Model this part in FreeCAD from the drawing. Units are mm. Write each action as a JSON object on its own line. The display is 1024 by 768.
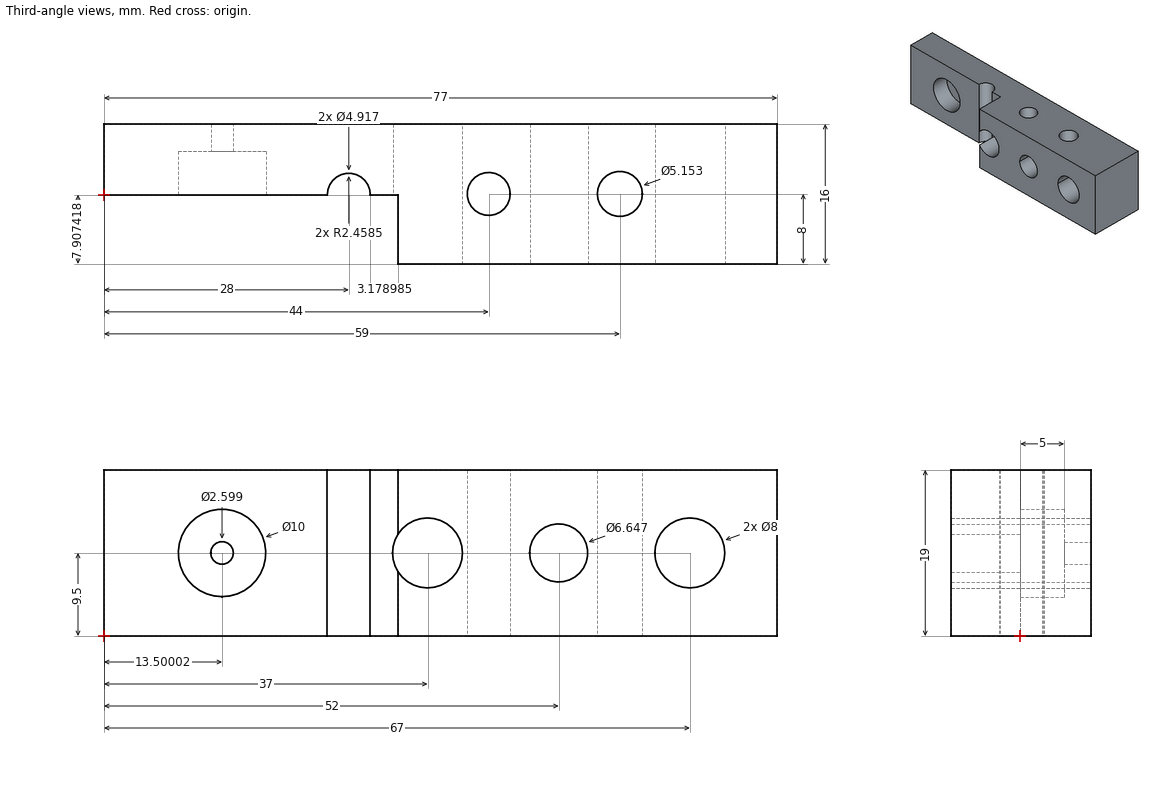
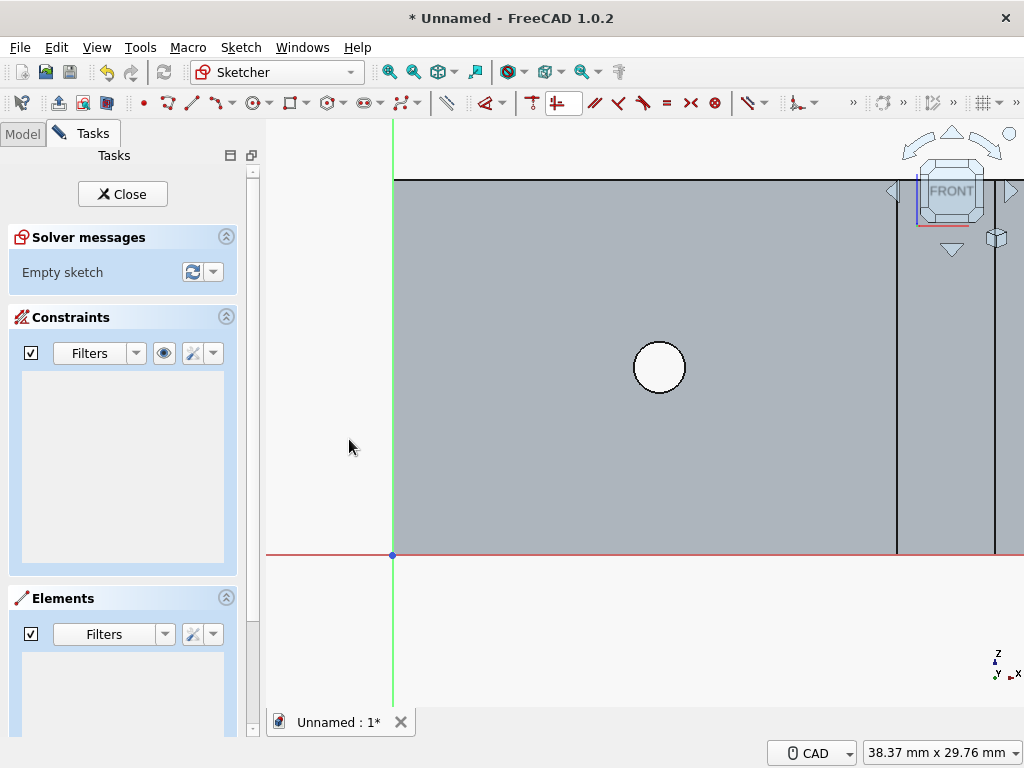
{"action": "key", "text": "g c"}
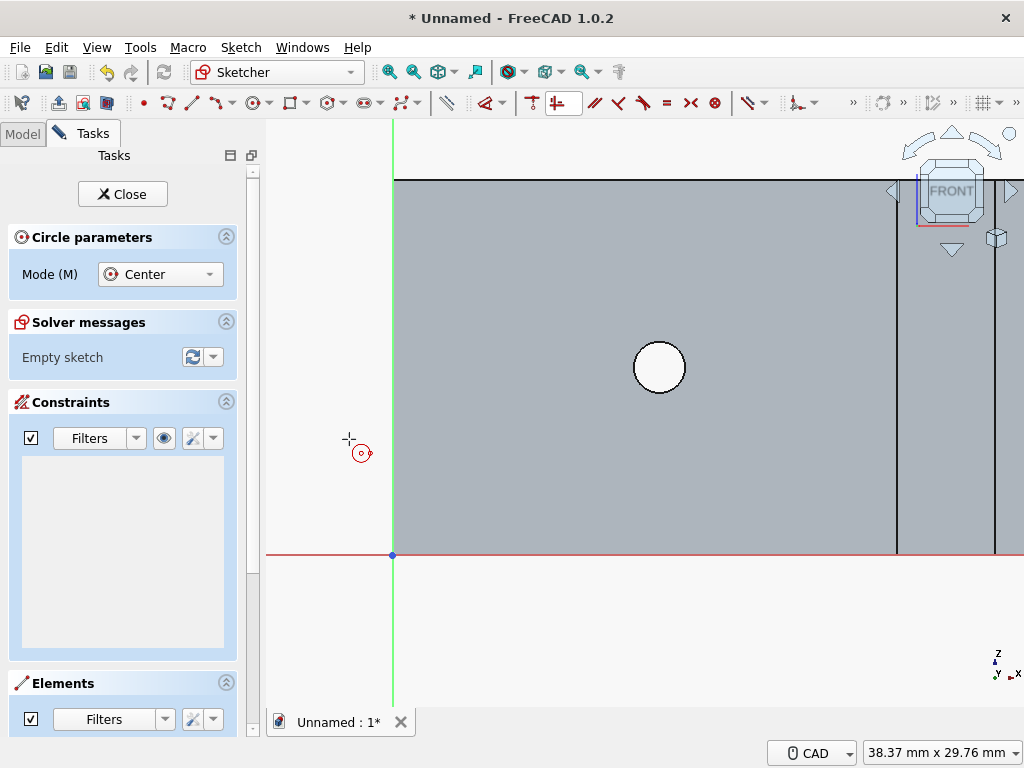
{"action": "left_click", "coordinate": [660, 367]}
{"action": "left_click", "coordinate": [729, 298]}
{"action": "key", "text": "Escape"}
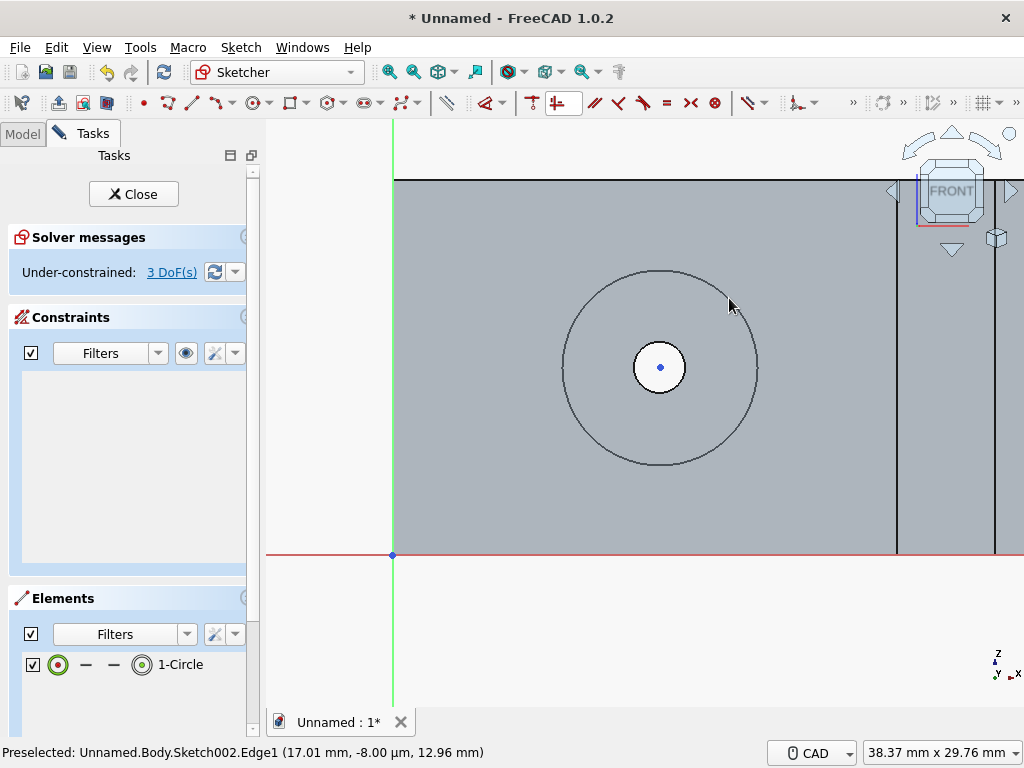
{"action": "left_click", "coordinate": [486, 104]}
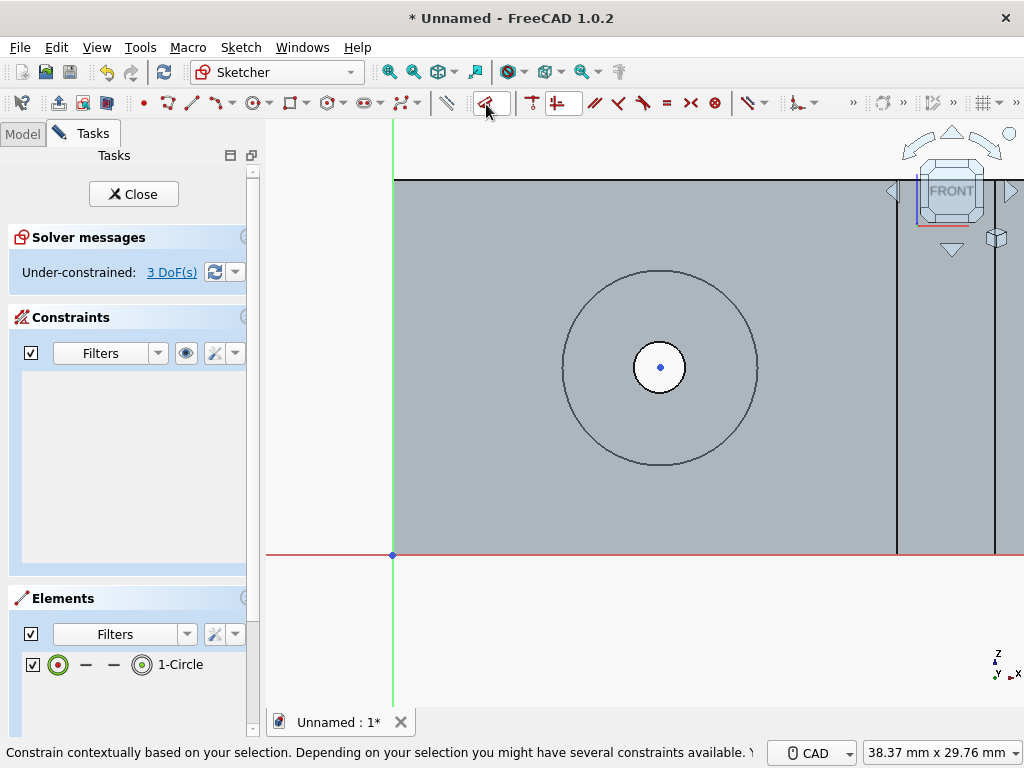
{"action": "left_click", "coordinate": [729, 299]}
{"action": "left_click", "coordinate": [752, 276]}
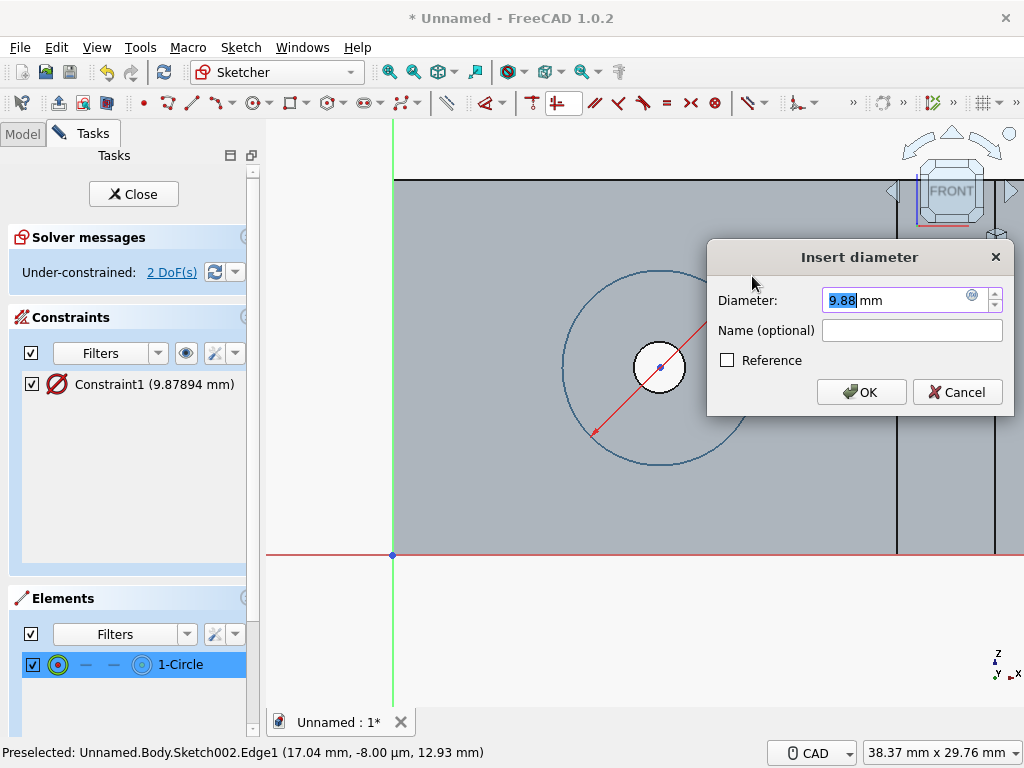
{"action": "type", "text": "10"}
{"action": "key", "text": "Return"}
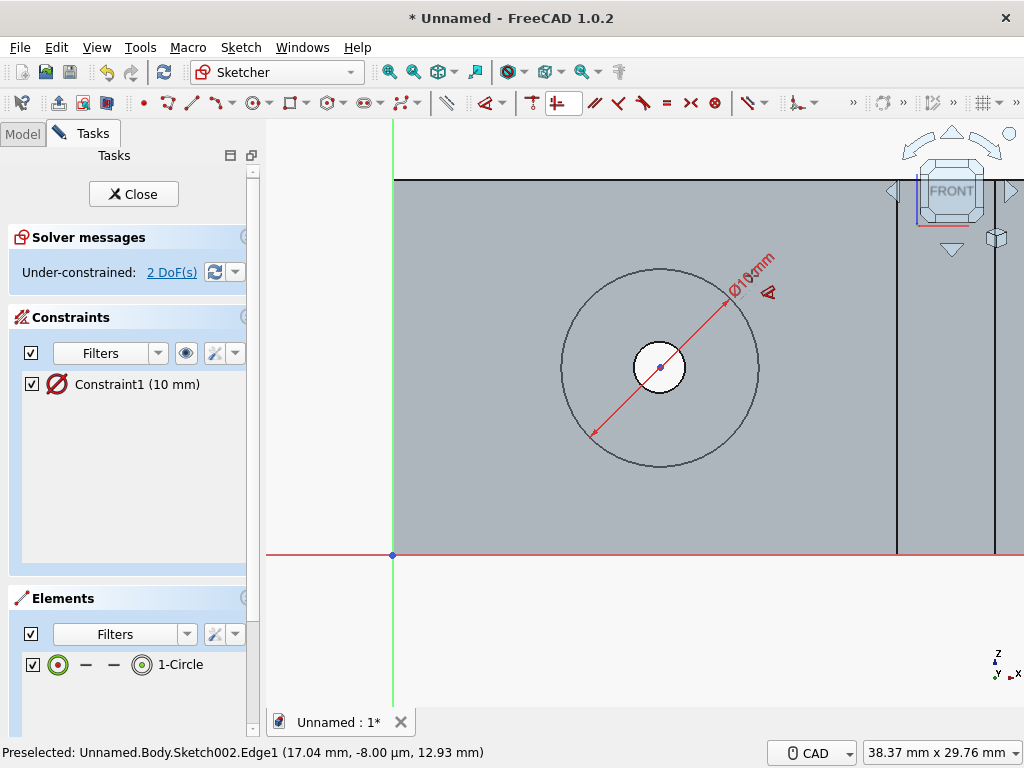
{"action": "left_click", "coordinate": [660, 368]}
{"action": "left_click", "coordinate": [359, 462]}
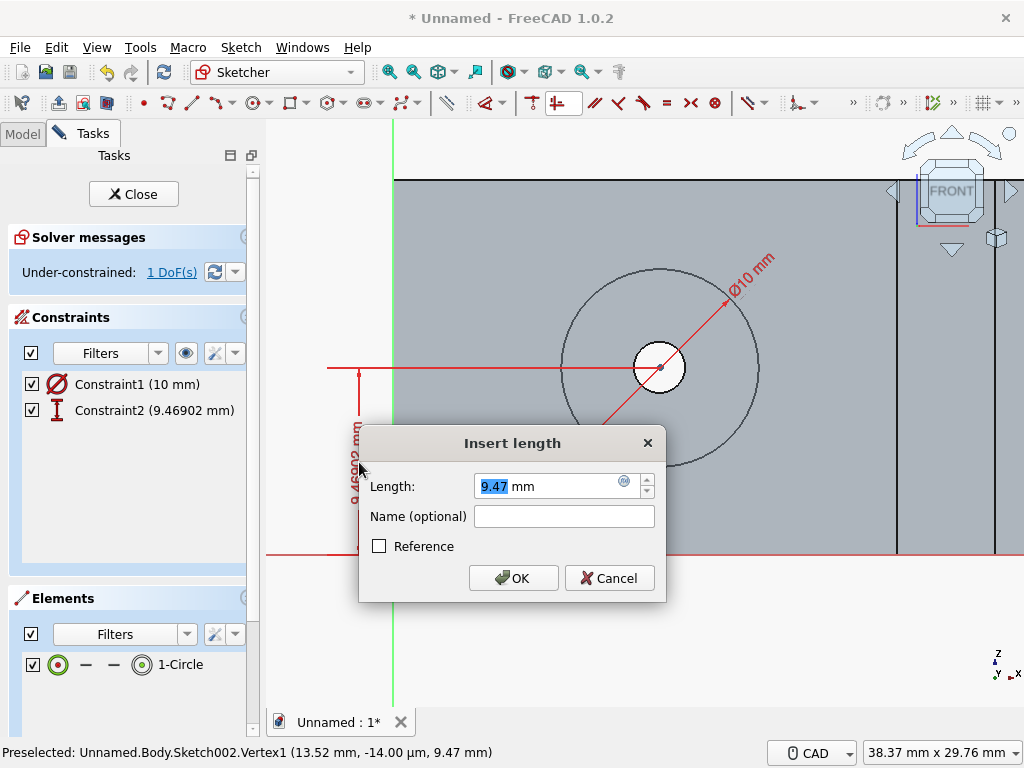
{"action": "type", "text": "9.5"}
{"action": "key", "text": "Return"}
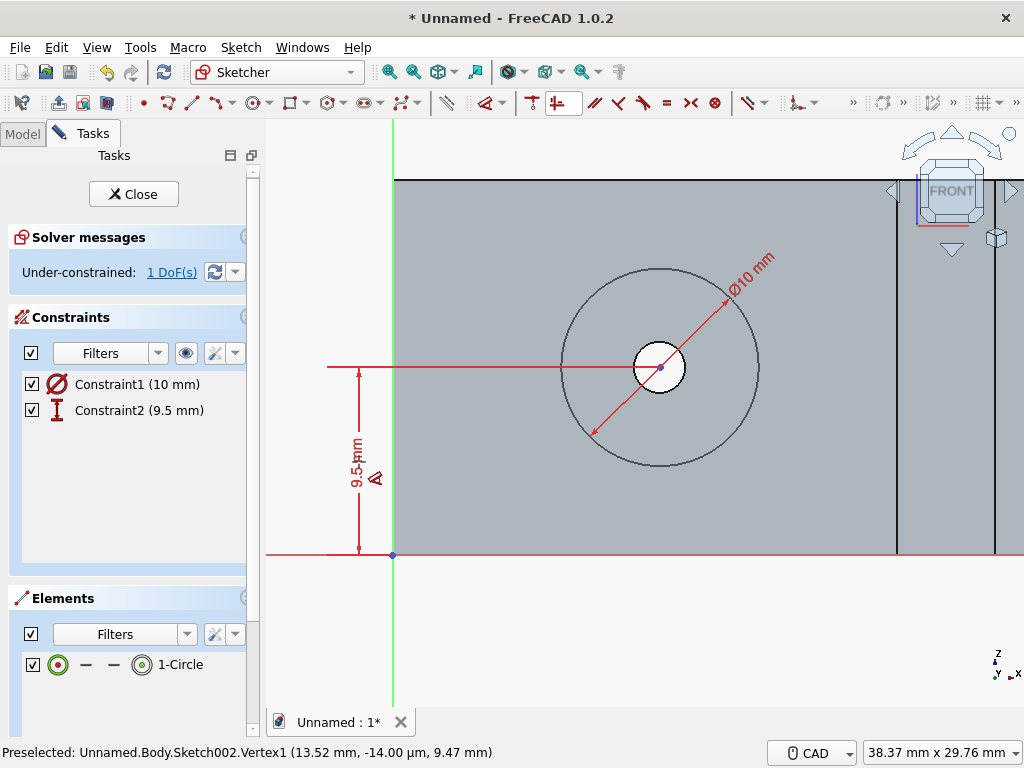
{"action": "left_click", "coordinate": [660, 367]}
{"action": "left_click", "coordinate": [526, 589]}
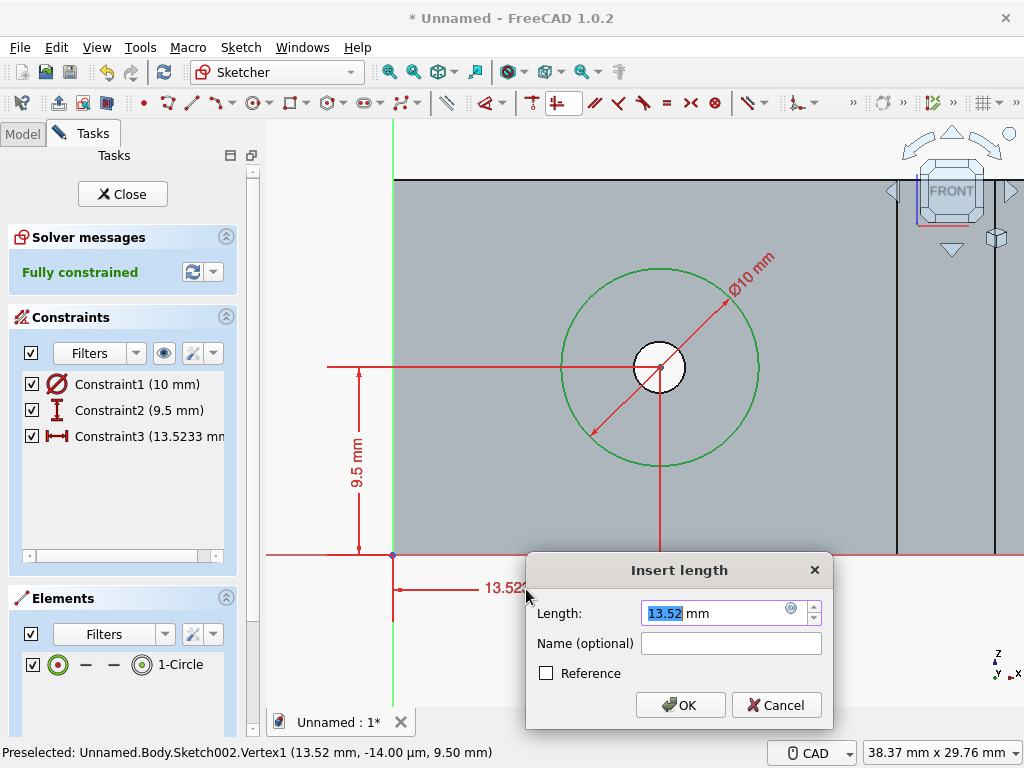
{"action": "type", "text": "13.50002"}
{"action": "key", "text": "Return"}
{"action": "key", "text": "Escape"}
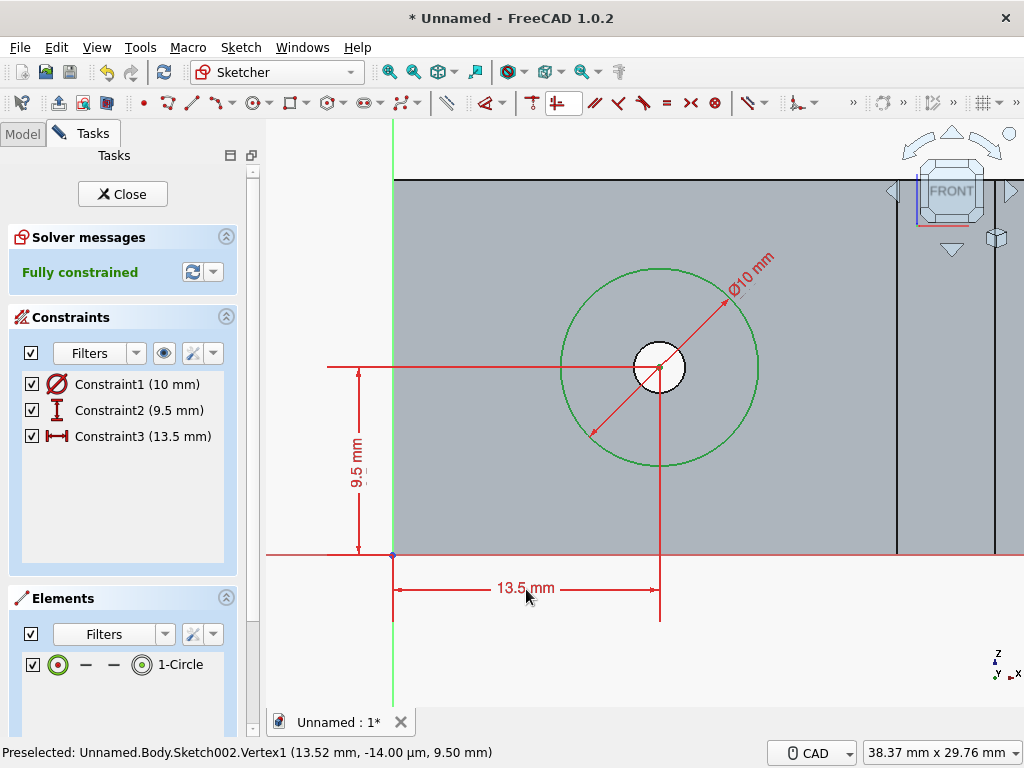
{"action": "left_click", "coordinate": [123, 194]}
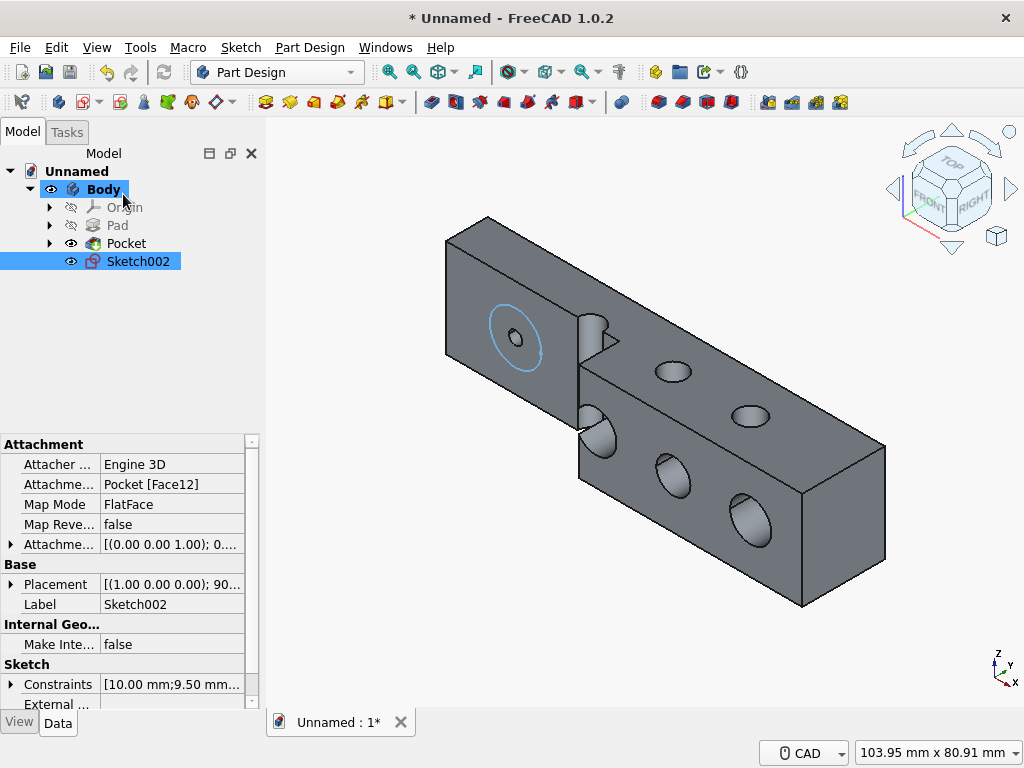
{"action": "left_click", "coordinate": [432, 102]}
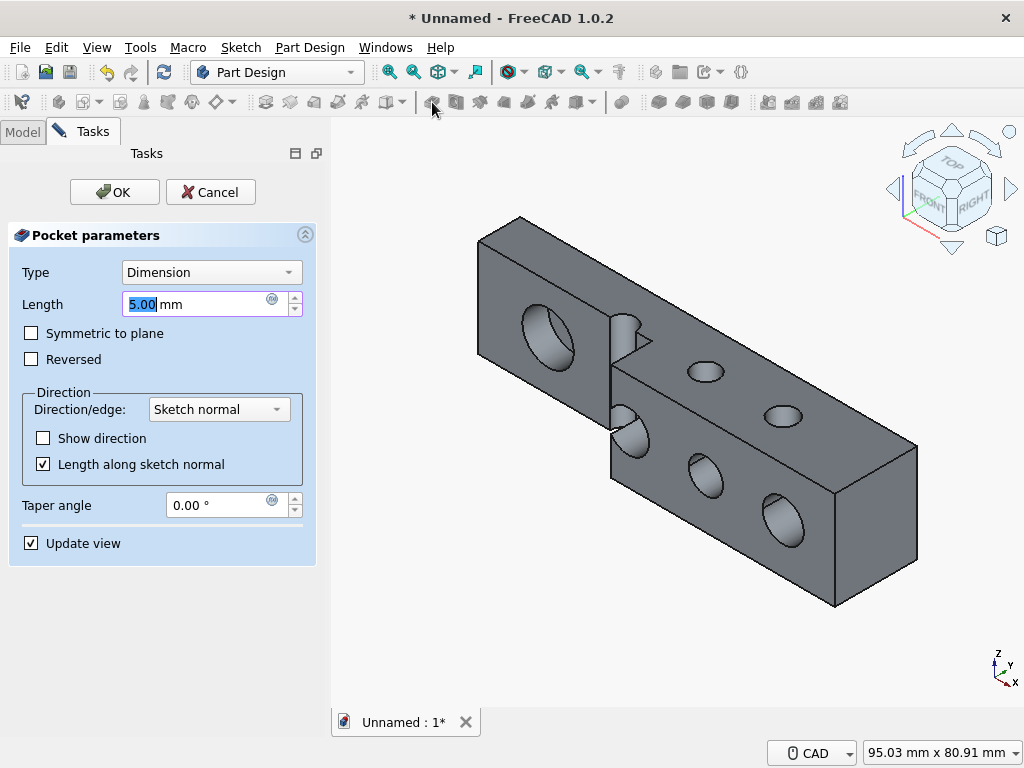
{"action": "type", "text": "5"}
{"action": "key", "text": "Tab"}